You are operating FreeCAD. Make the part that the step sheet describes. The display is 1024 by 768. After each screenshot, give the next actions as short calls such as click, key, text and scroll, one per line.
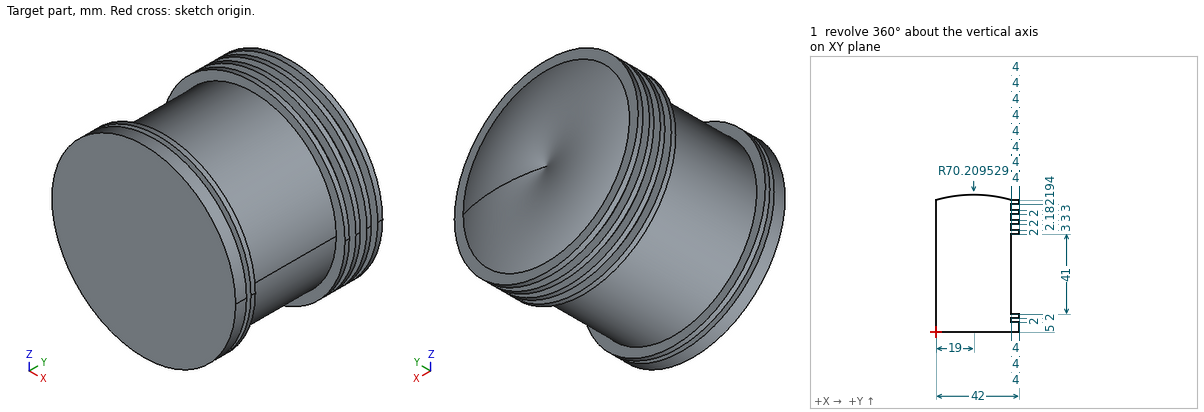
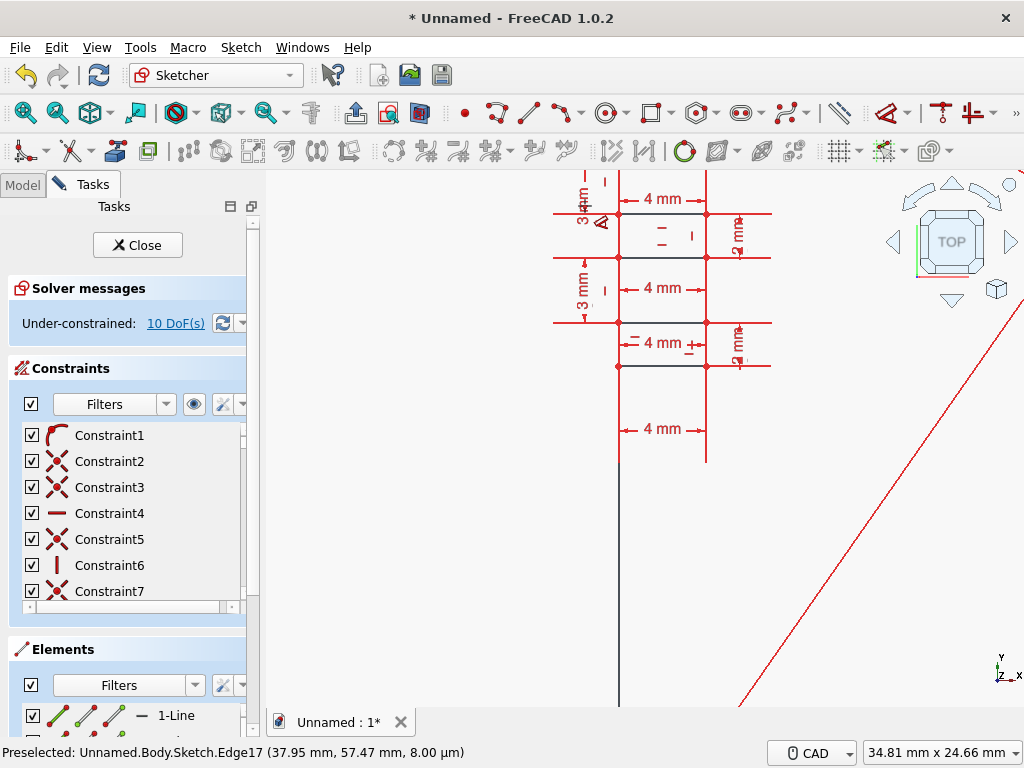
scroll(683, 355, down, 7)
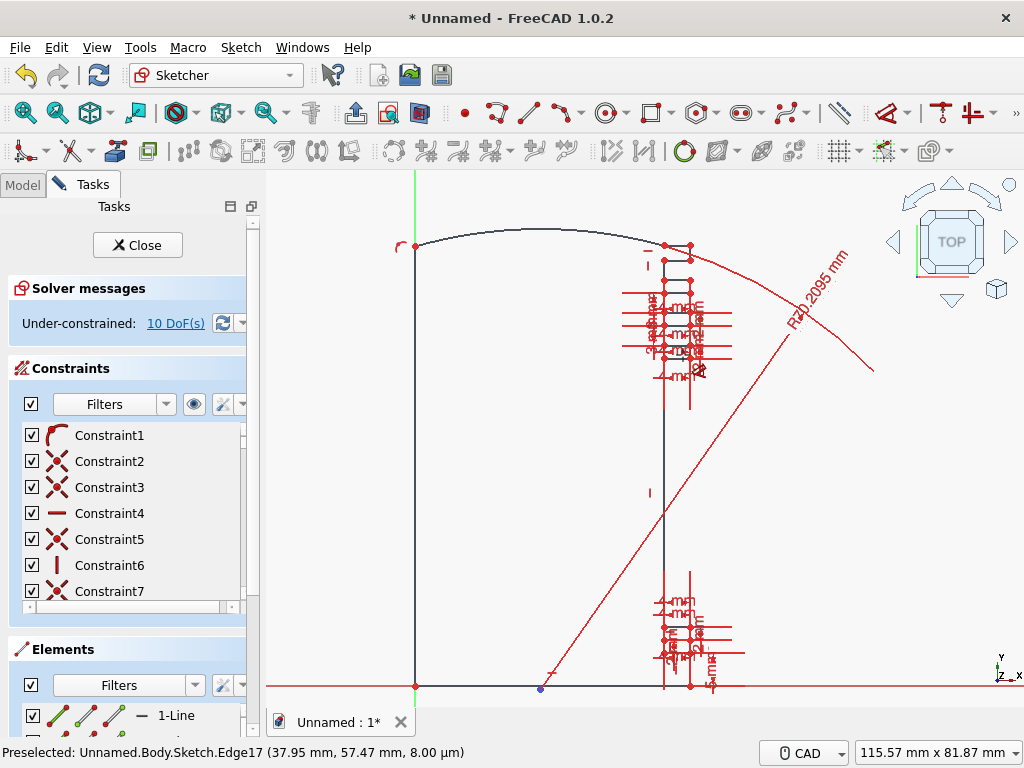
scroll(674, 304, up, 4)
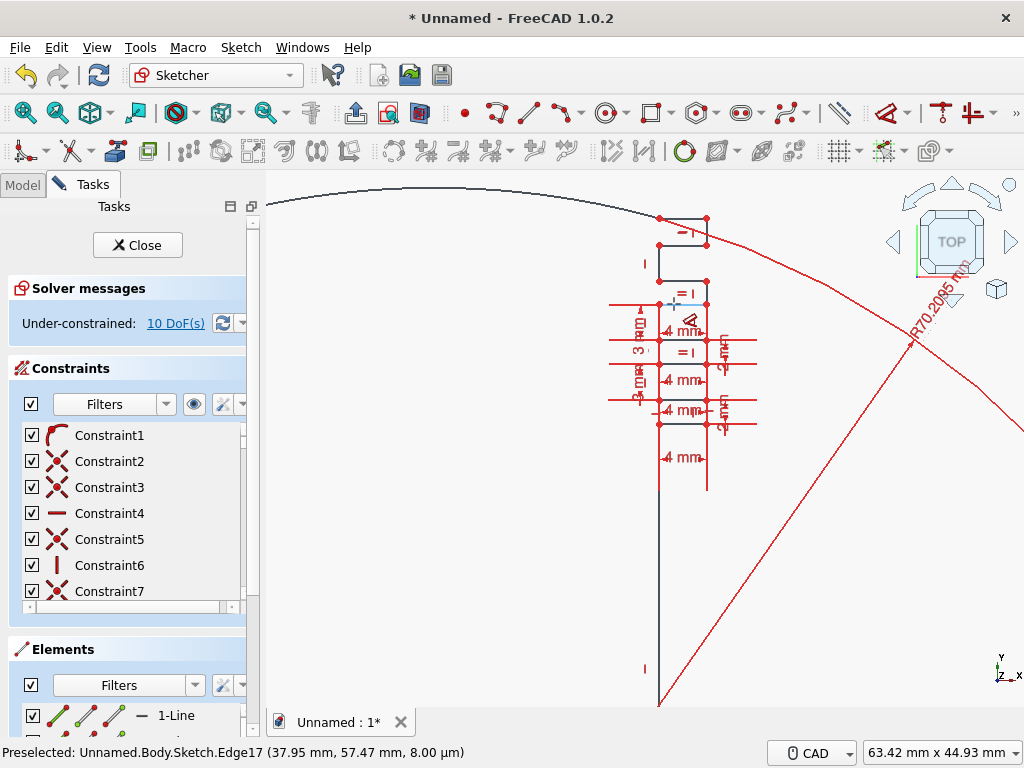
click(673, 305)
click(683, 199)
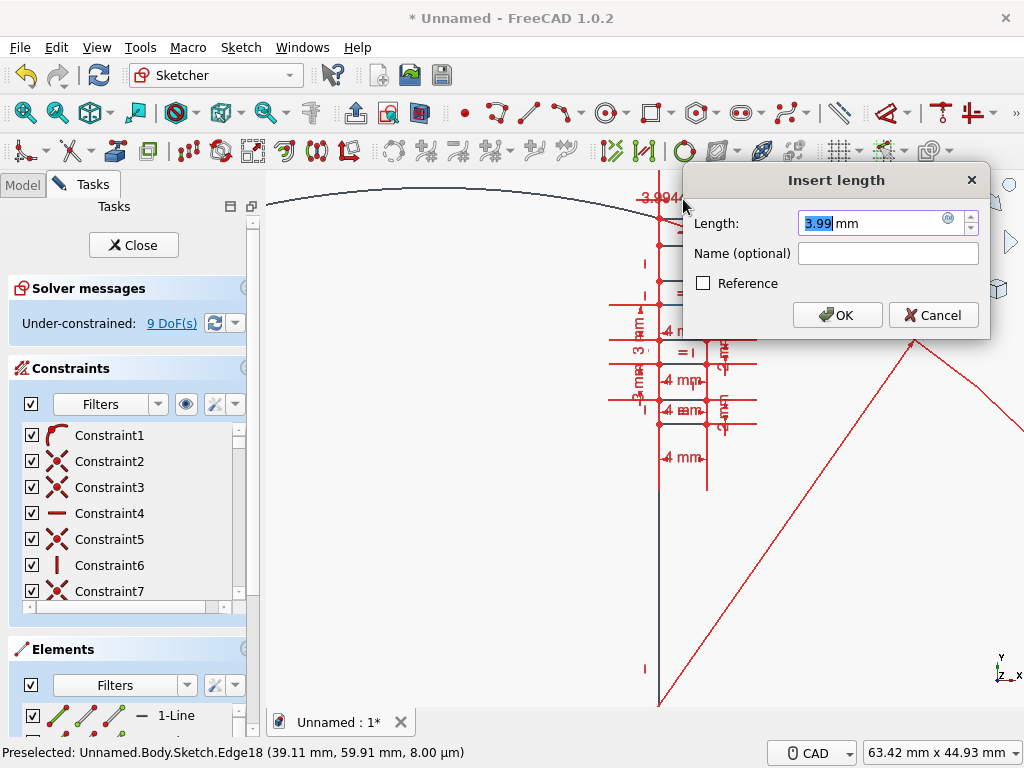
text(4)
key(Return)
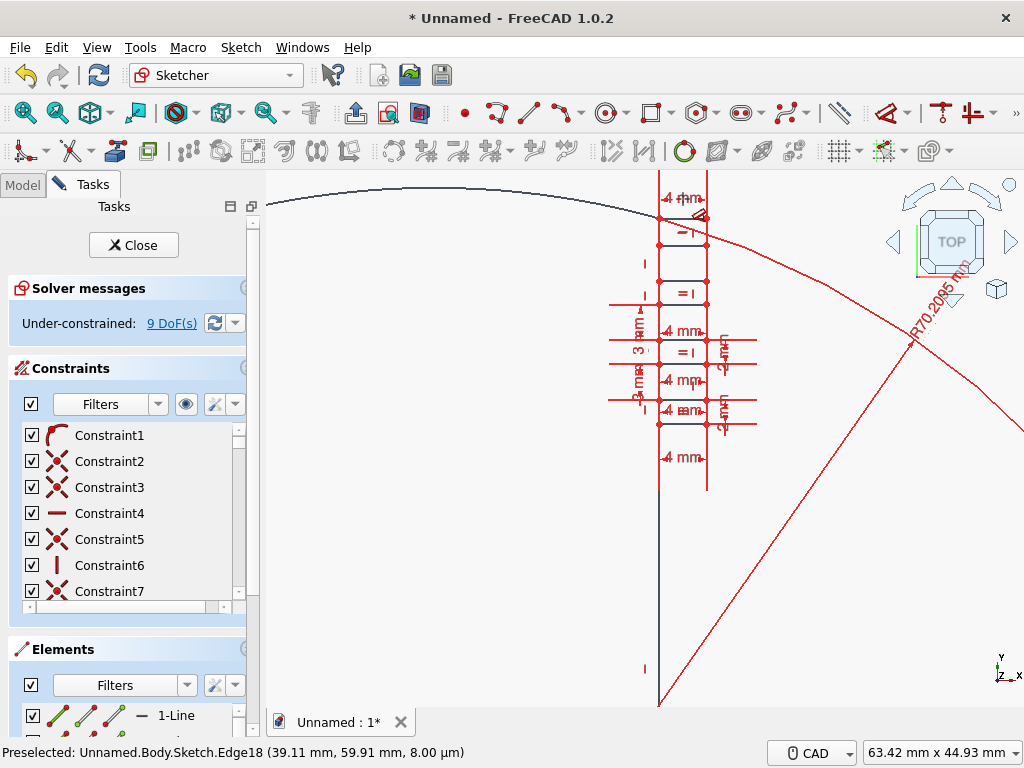
scroll(707, 295, up, 3)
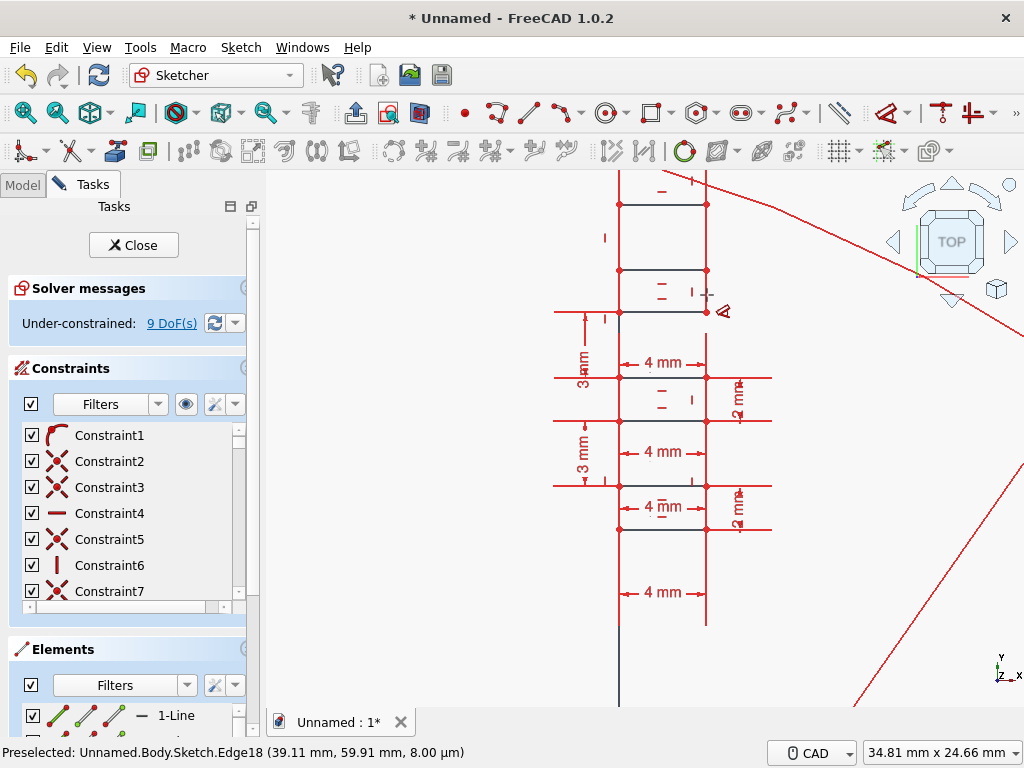
click(706, 295)
click(740, 291)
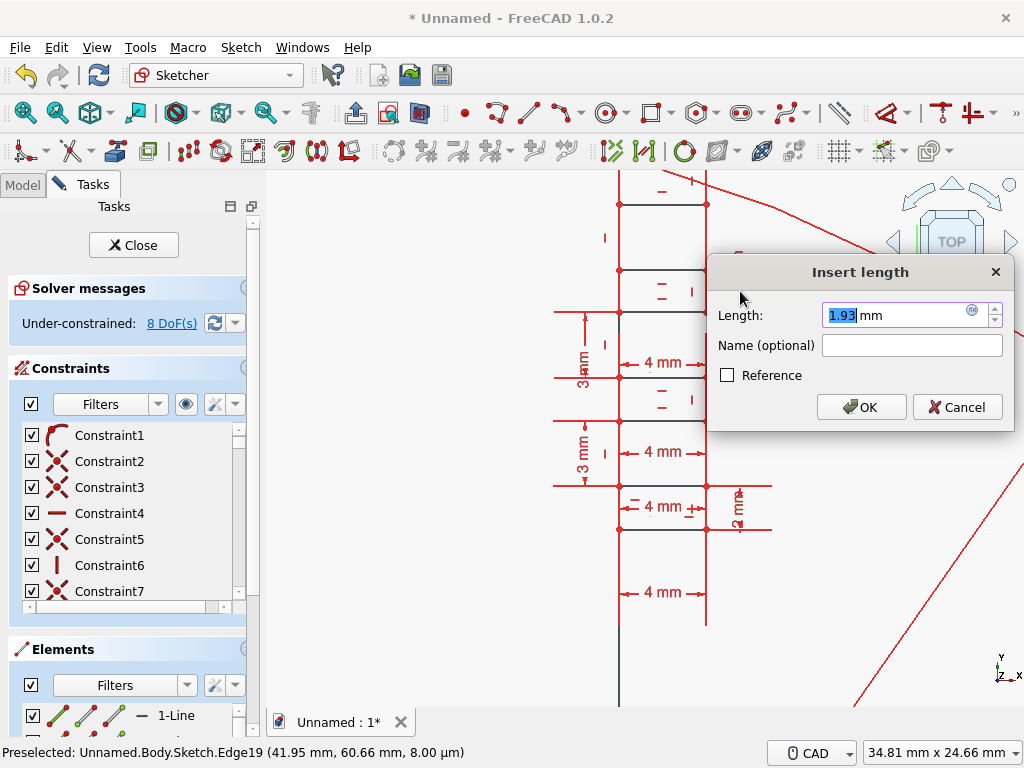
text(2)
key(Return)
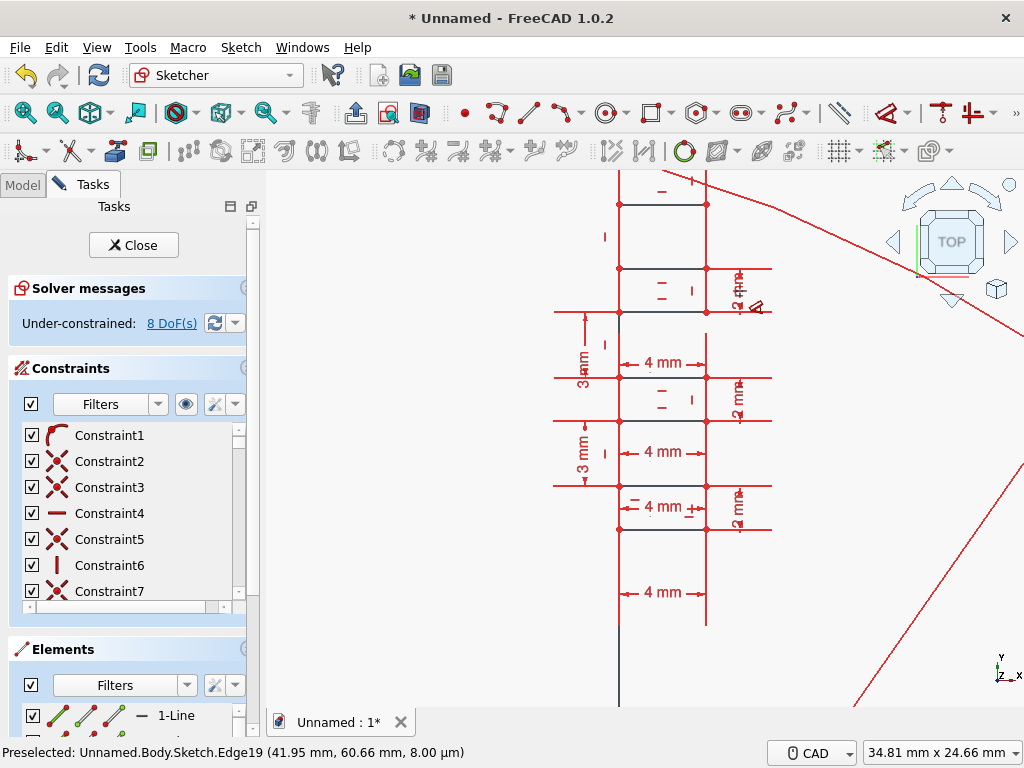
click(680, 269)
click(663, 235)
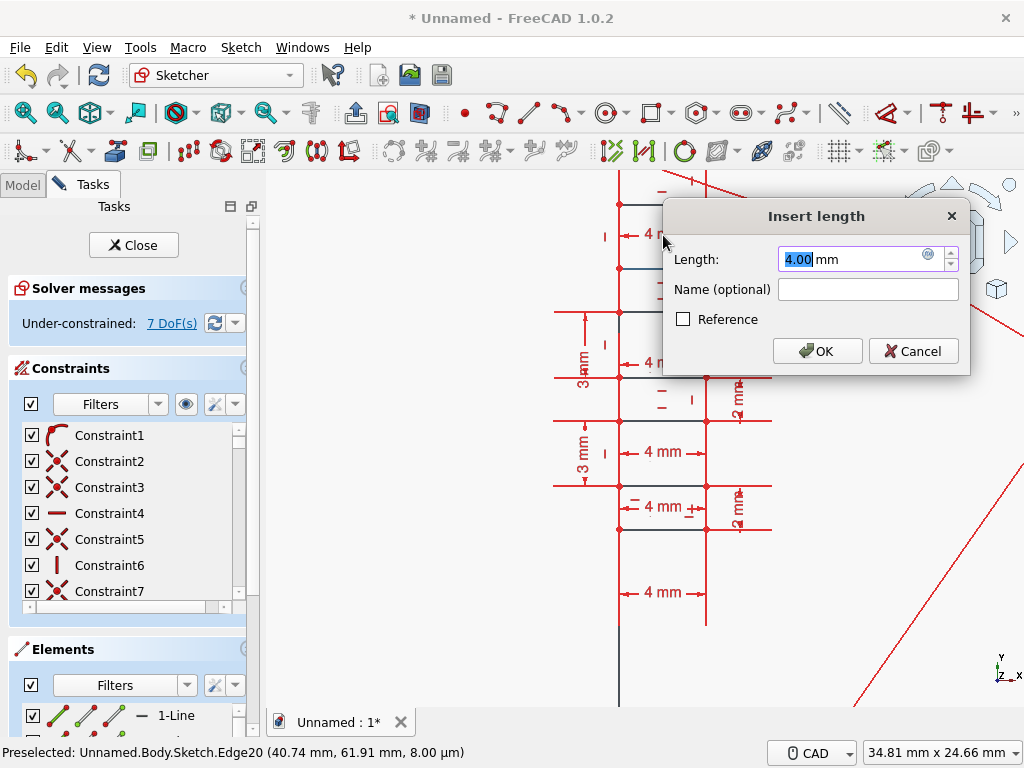
text(4)
key(Return)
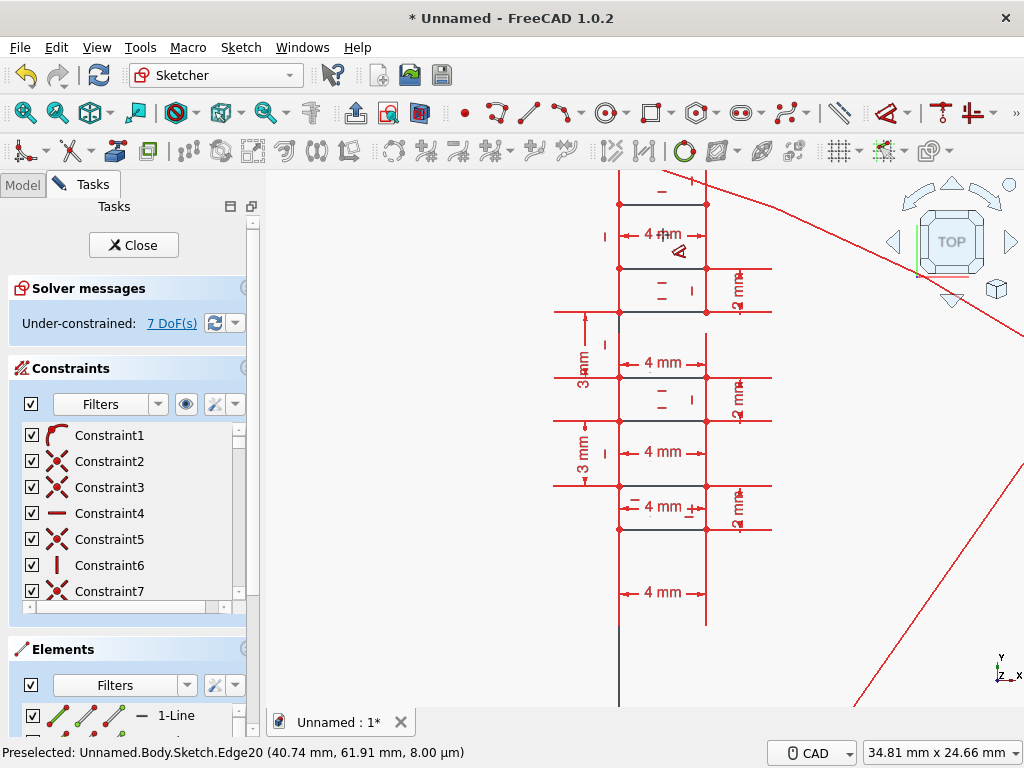
click(619, 250)
click(585, 237)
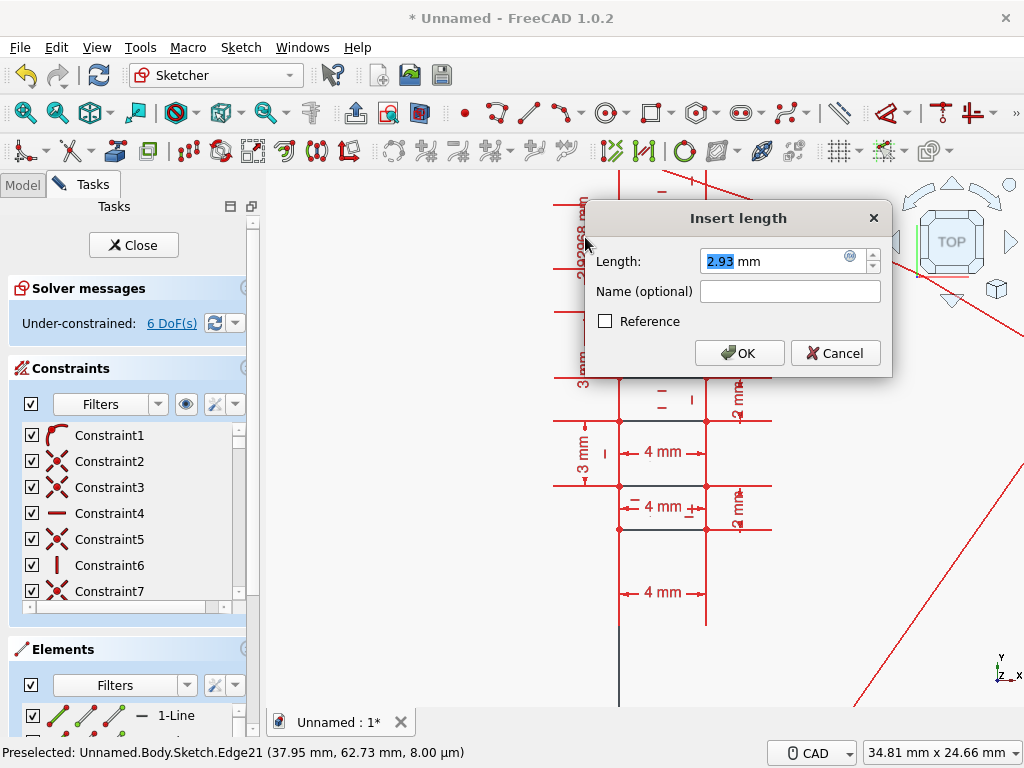
text(3)
key(Return)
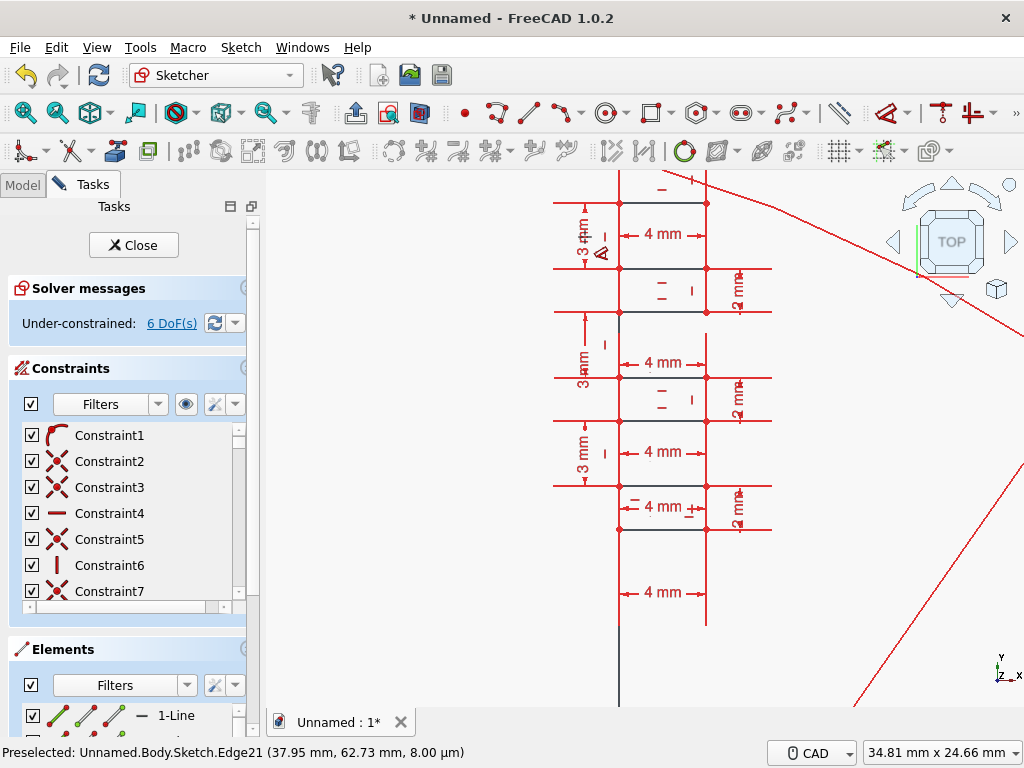
click(645, 203)
click(663, 285)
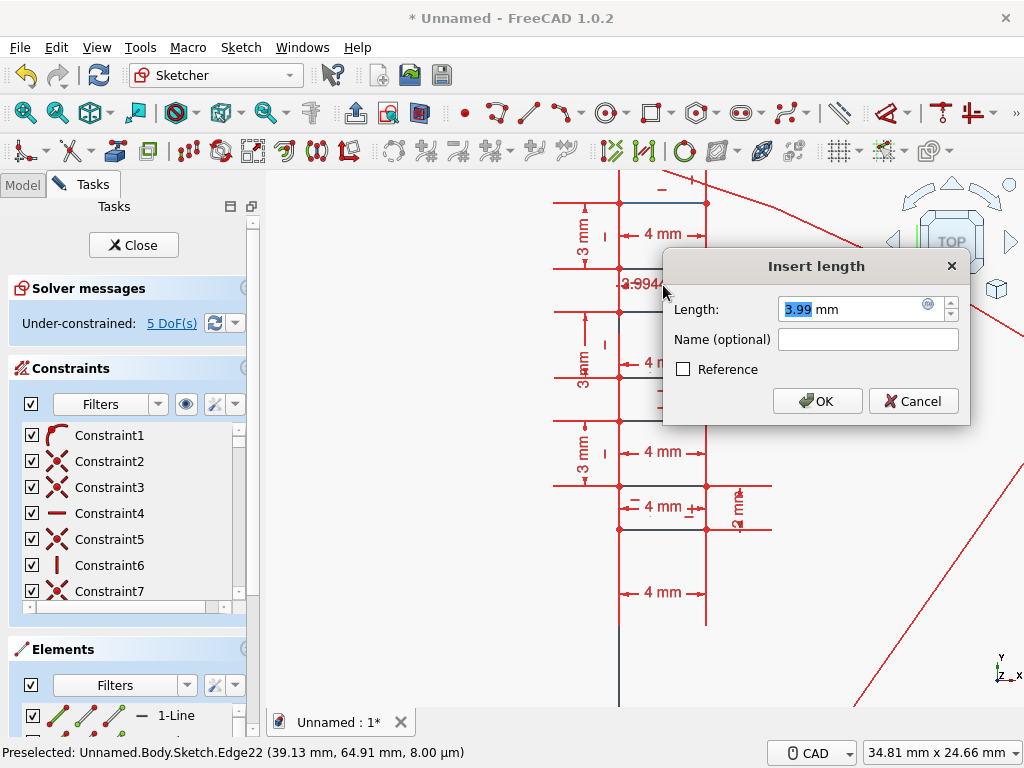
text(4)
key(Return)